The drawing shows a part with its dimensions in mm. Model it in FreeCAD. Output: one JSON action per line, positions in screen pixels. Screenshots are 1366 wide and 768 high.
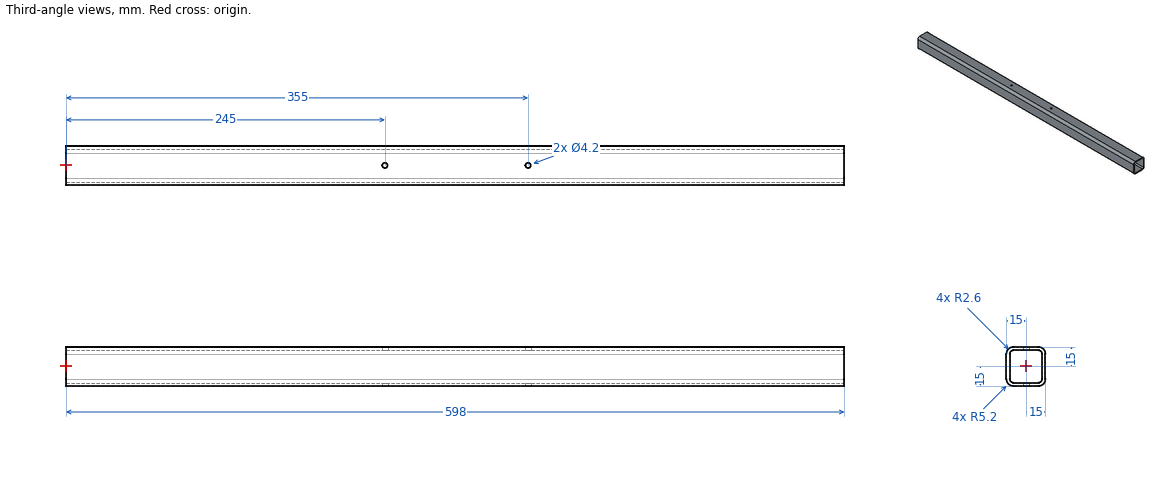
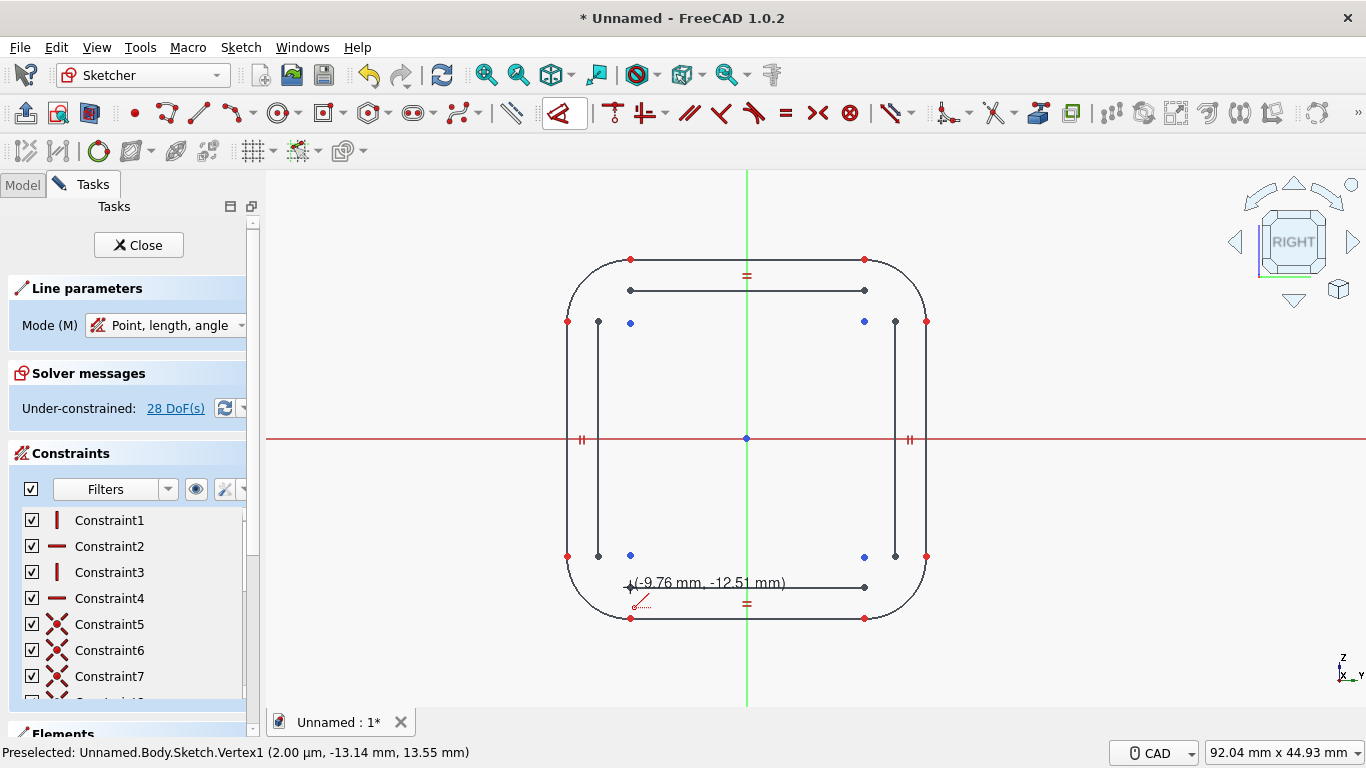
{"action": "key", "text": "g 3 a"}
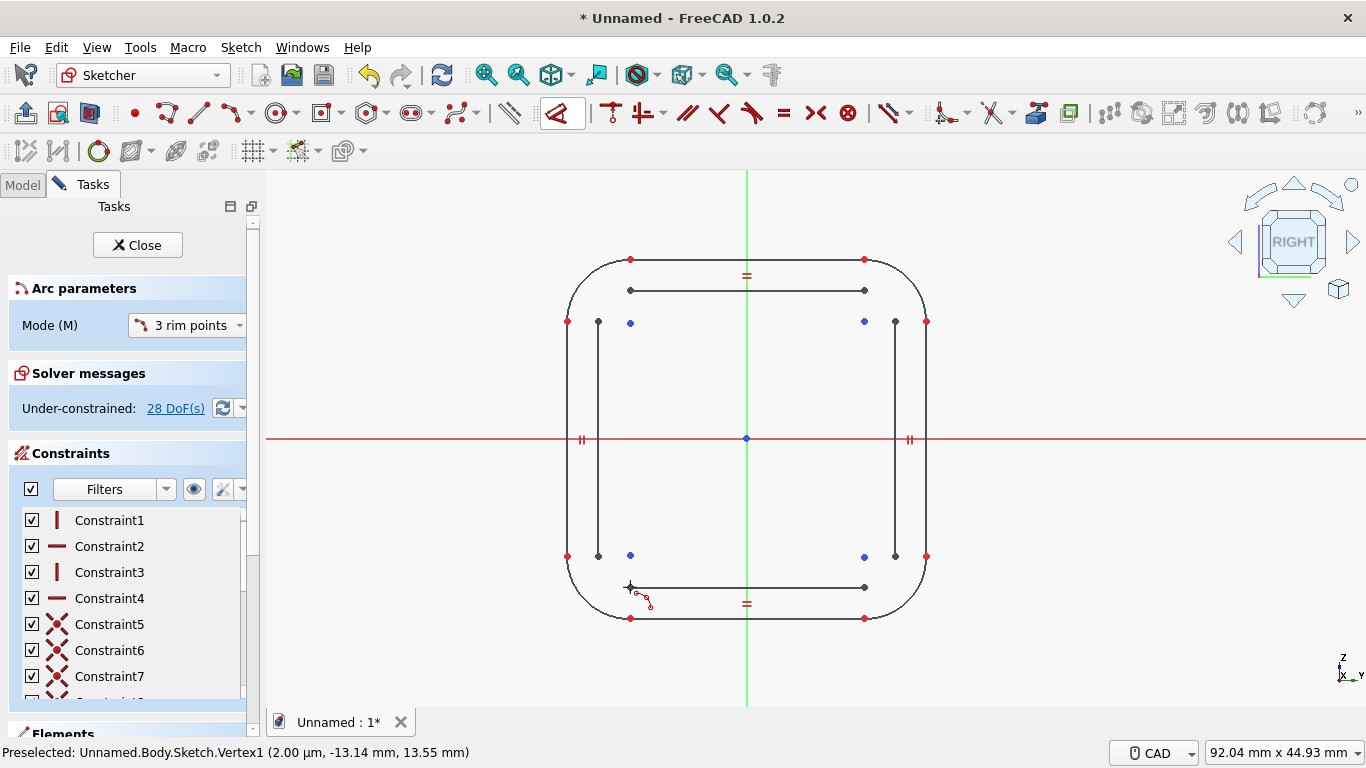
{"action": "left_click", "coordinate": [598, 322]}
{"action": "left_click", "coordinate": [630, 291]}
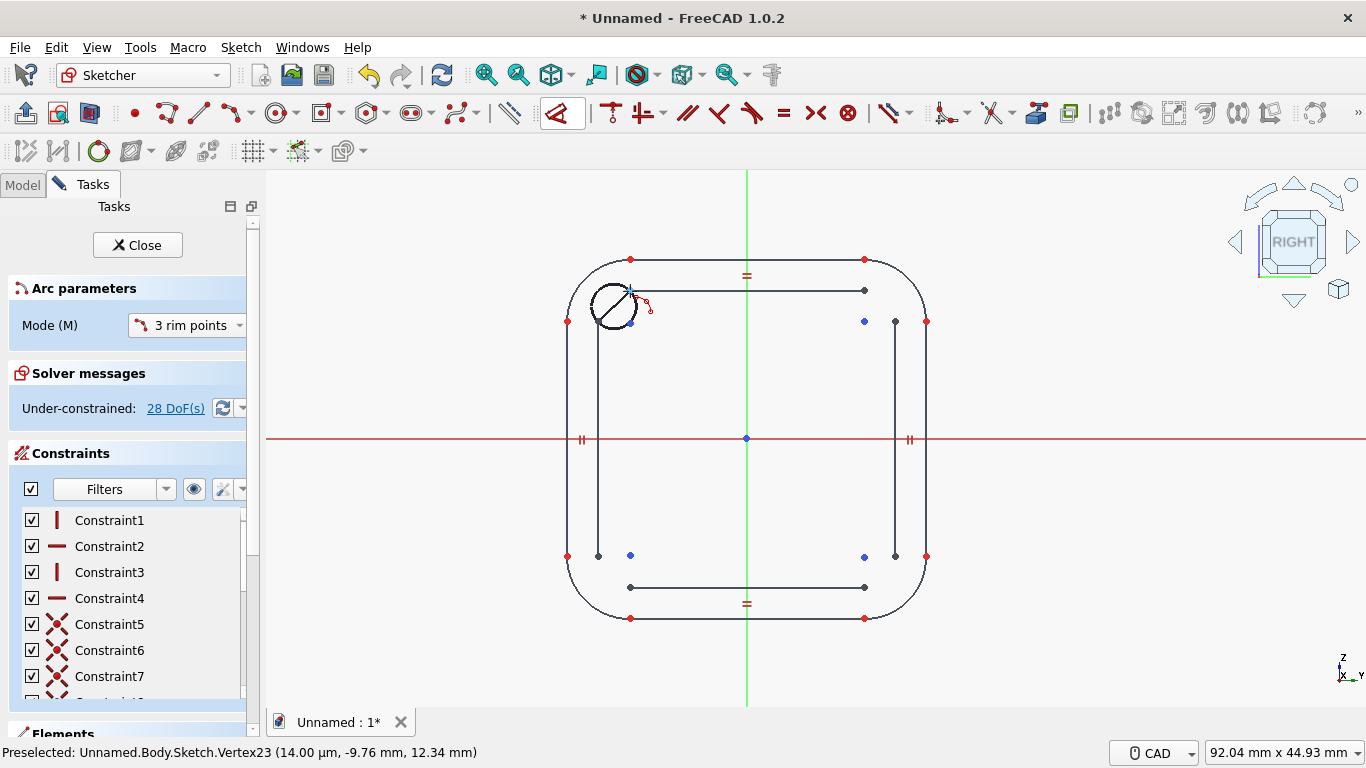
{"action": "scroll", "coordinate": [608, 299], "scroll_direction": "up", "scroll_amount": 3}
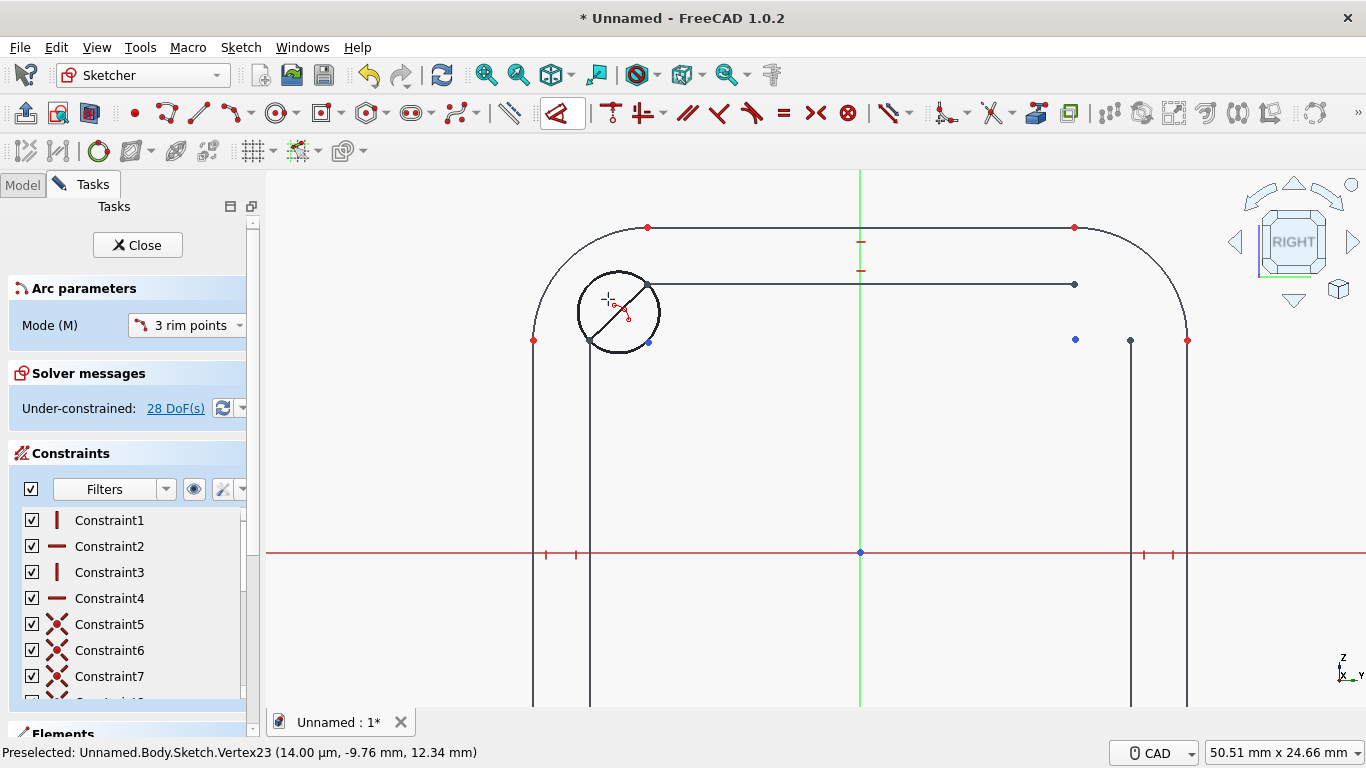
{"action": "left_click", "coordinate": [607, 300]}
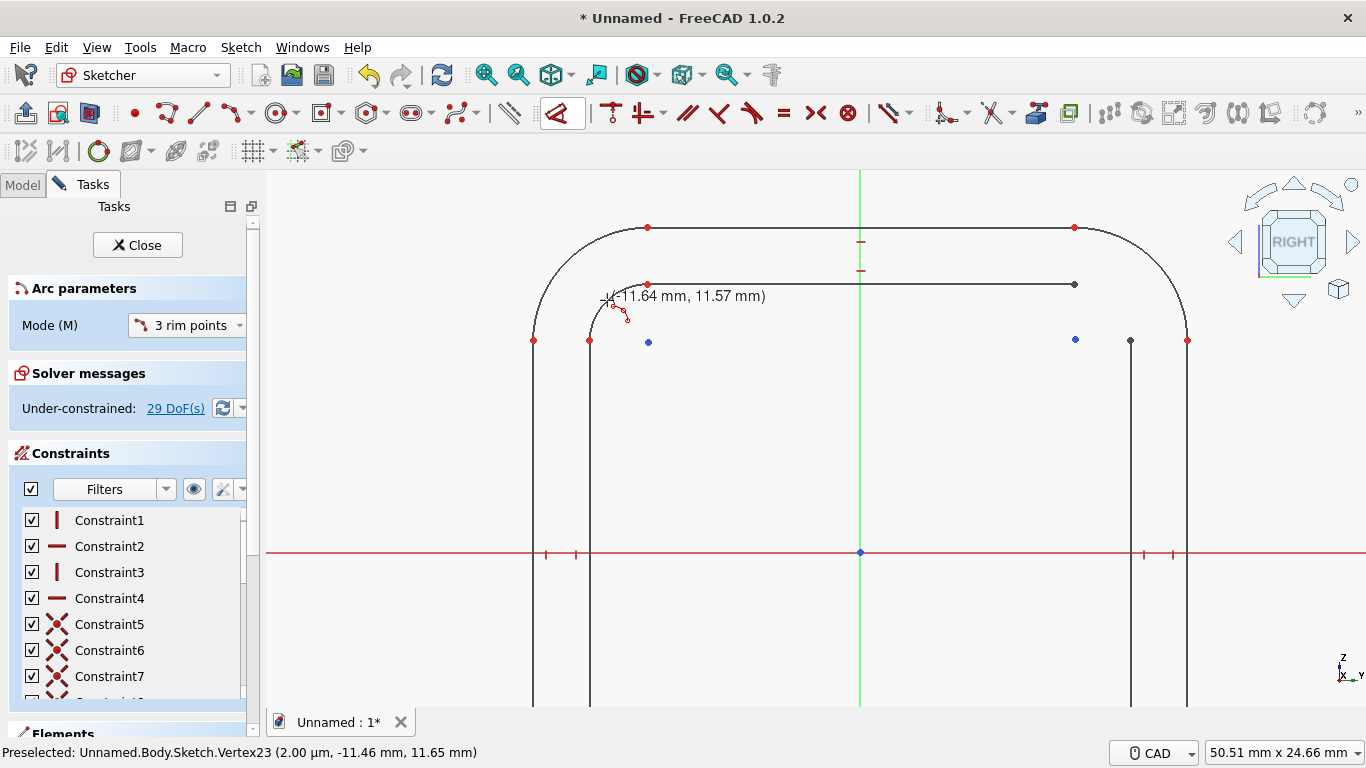
{"action": "left_click", "coordinate": [1074, 284]}
{"action": "left_click", "coordinate": [1131, 341]}
{"action": "left_click", "coordinate": [1114, 300]}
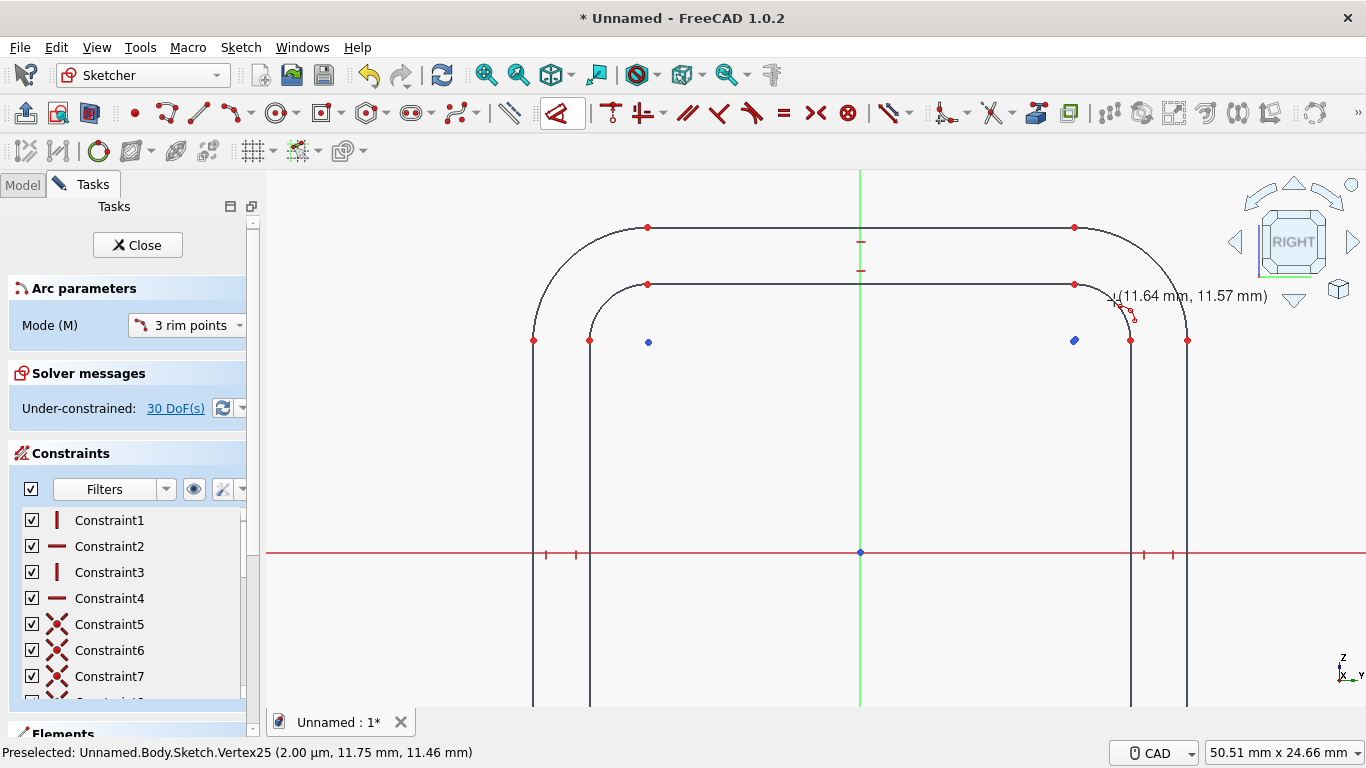
{"action": "scroll", "coordinate": [610, 299], "scroll_direction": "down", "scroll_amount": 3}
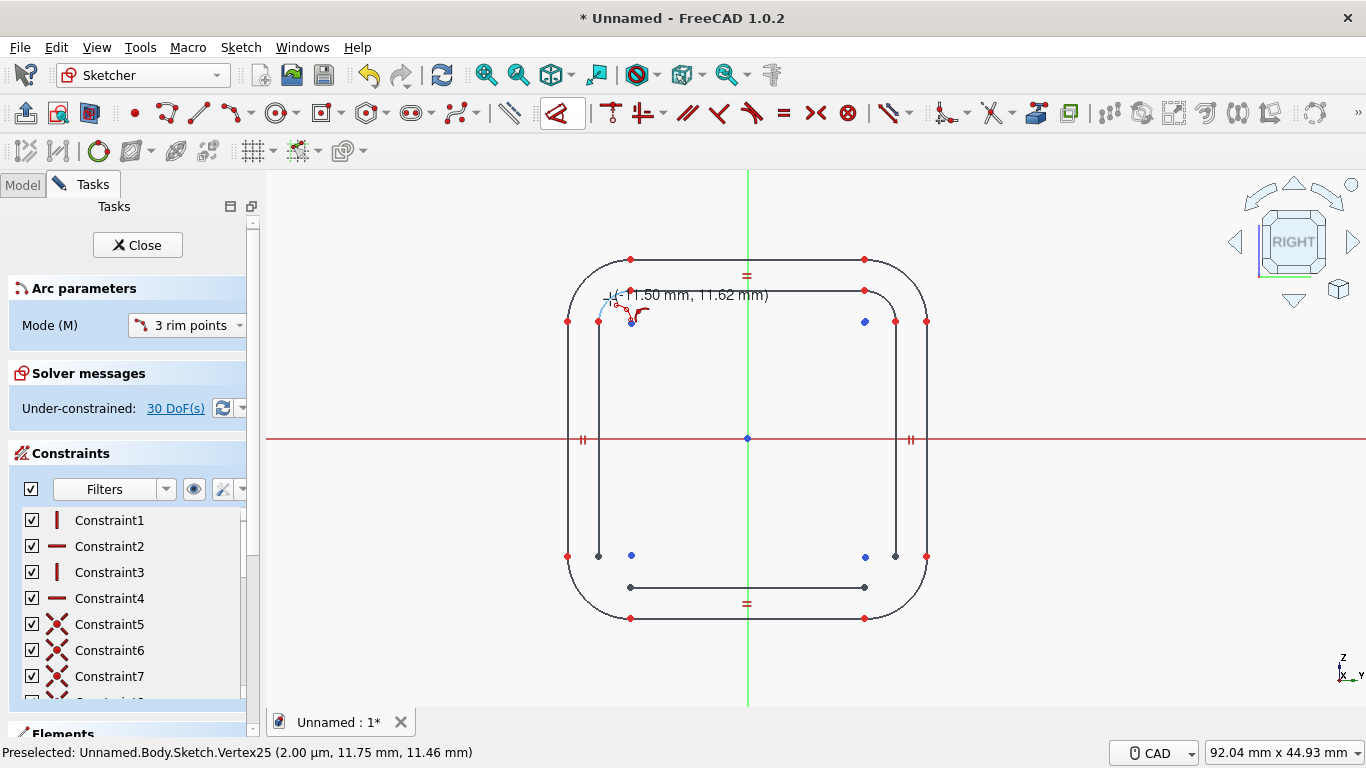
{"action": "left_click", "coordinate": [896, 557]}
{"action": "left_click", "coordinate": [865, 588]}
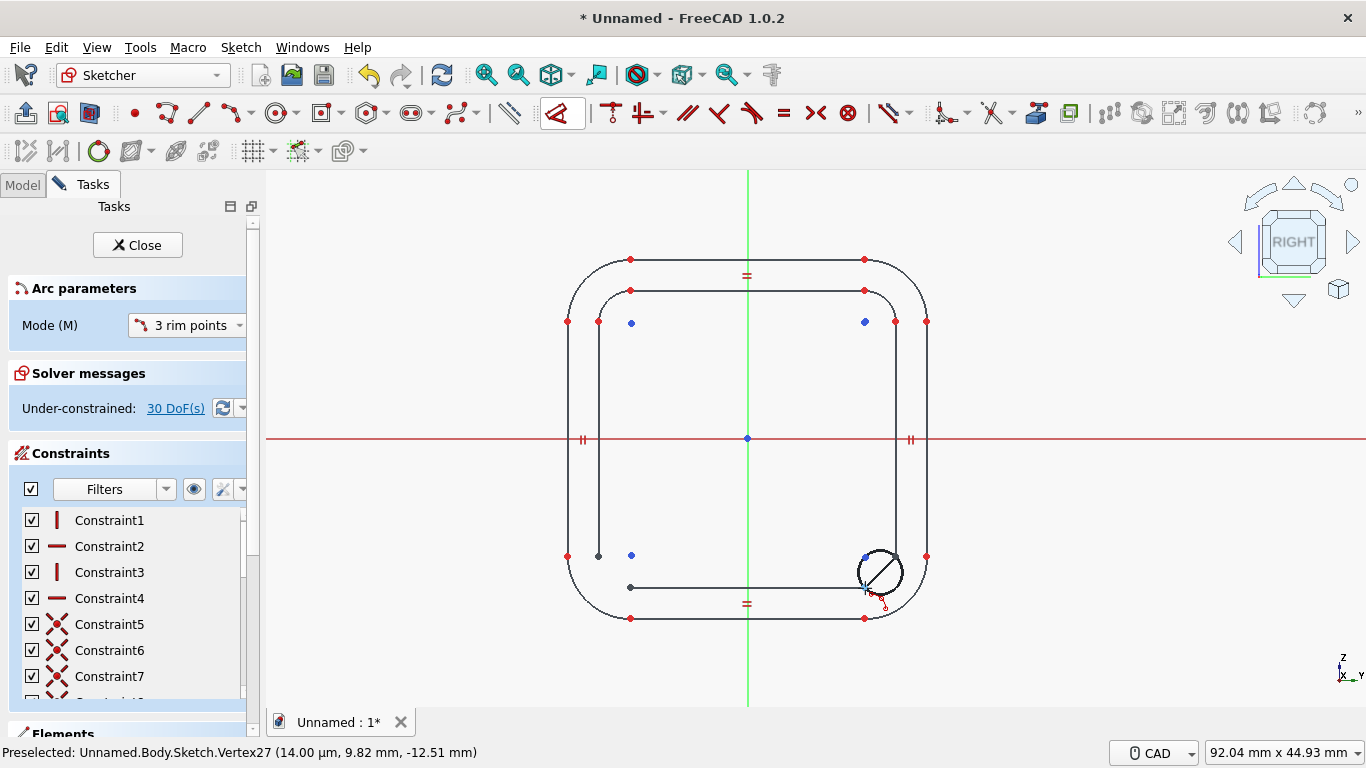
{"action": "scroll", "coordinate": [887, 578], "scroll_direction": "up", "scroll_amount": 3}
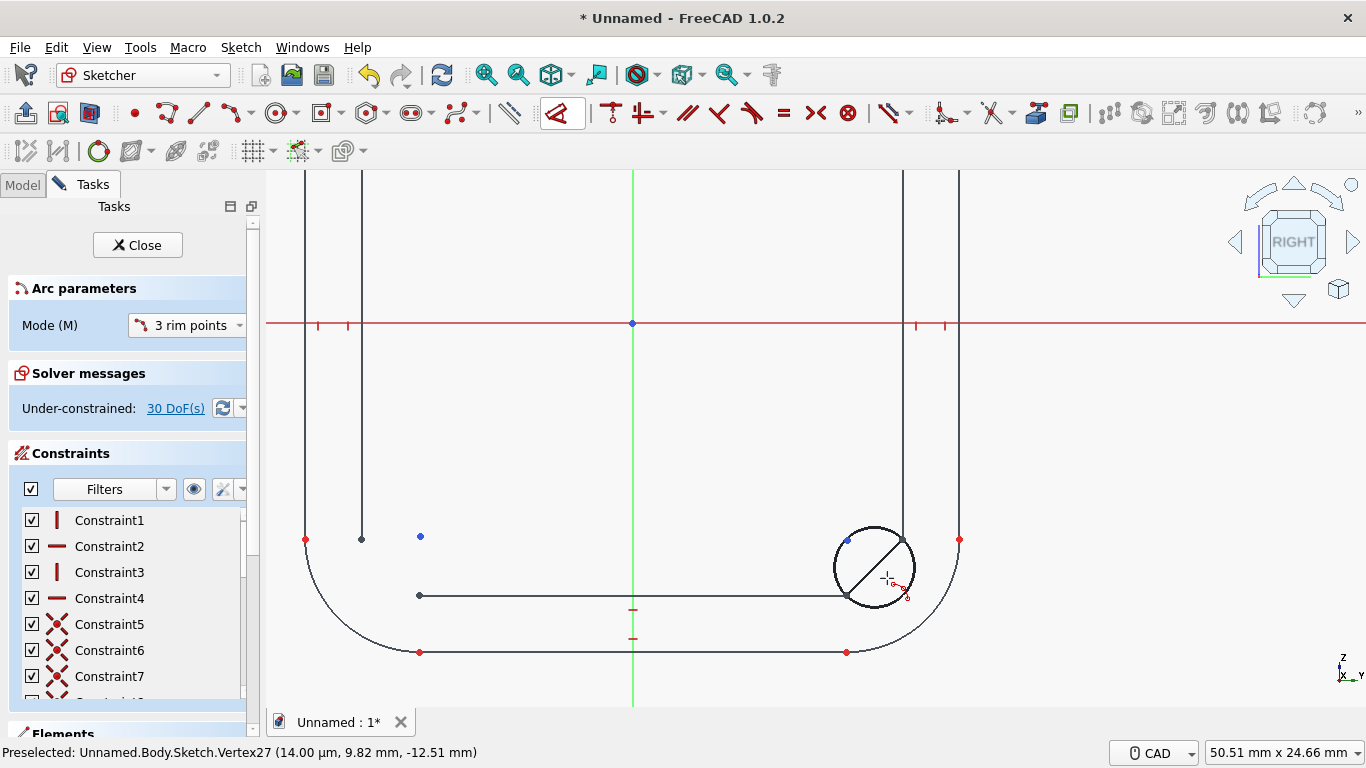
{"action": "left_click", "coordinate": [886, 577]}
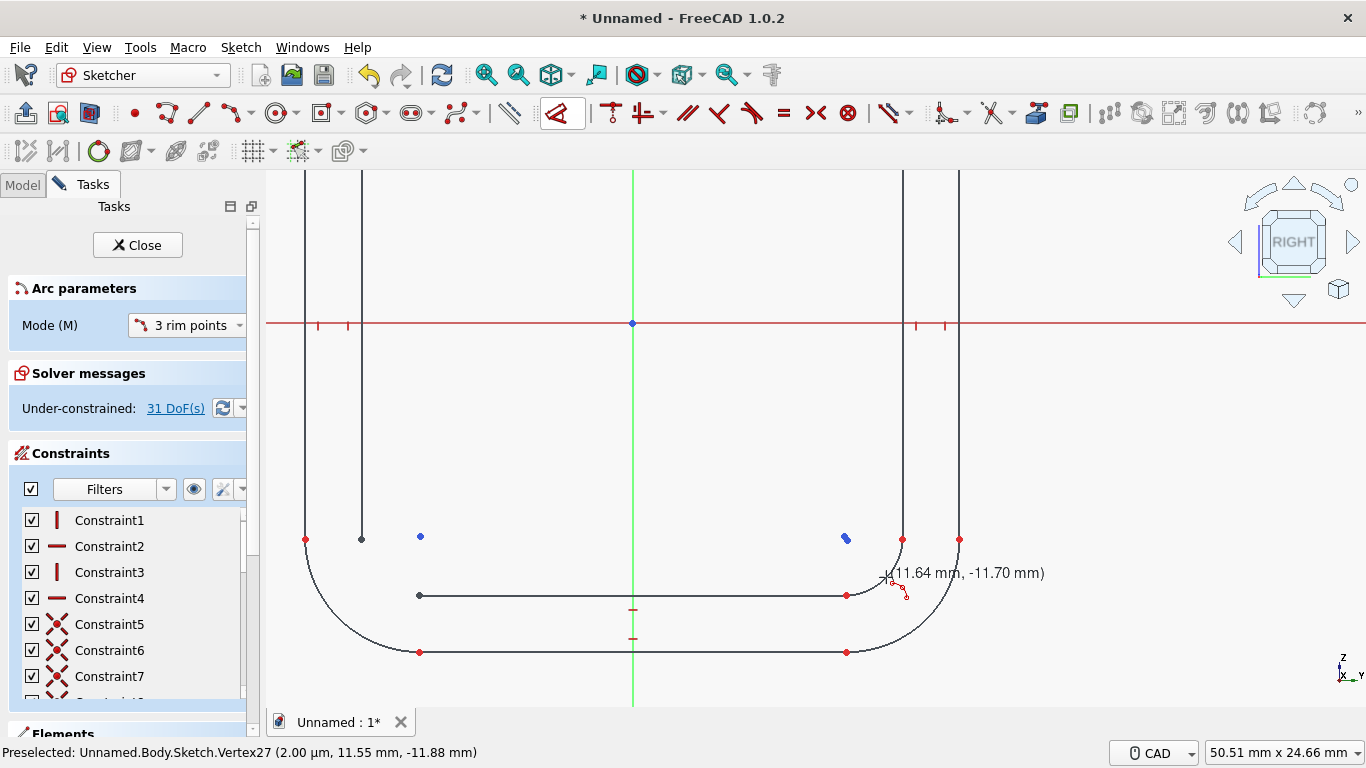
{"action": "left_click", "coordinate": [420, 596]}
{"action": "left_click", "coordinate": [362, 539]}
{"action": "left_click", "coordinate": [379, 577]}
{"action": "key", "text": "Escape"}